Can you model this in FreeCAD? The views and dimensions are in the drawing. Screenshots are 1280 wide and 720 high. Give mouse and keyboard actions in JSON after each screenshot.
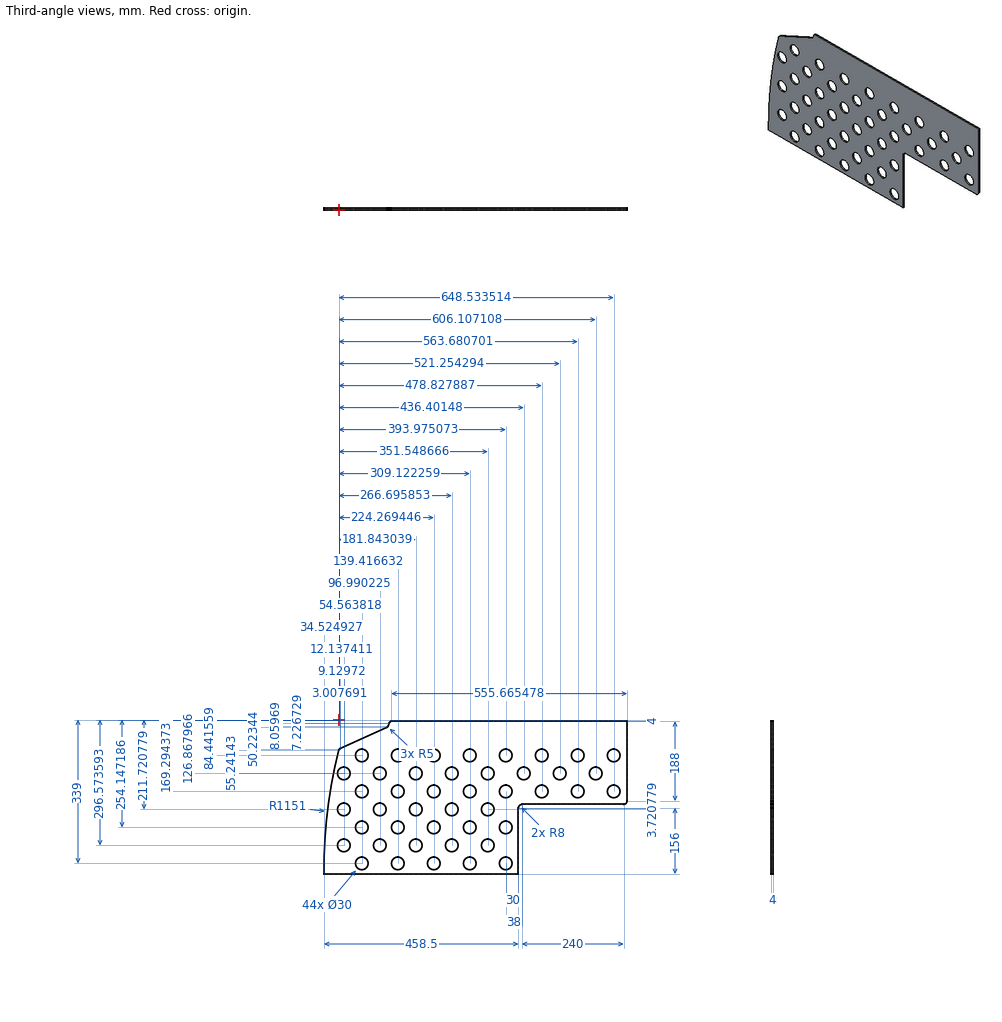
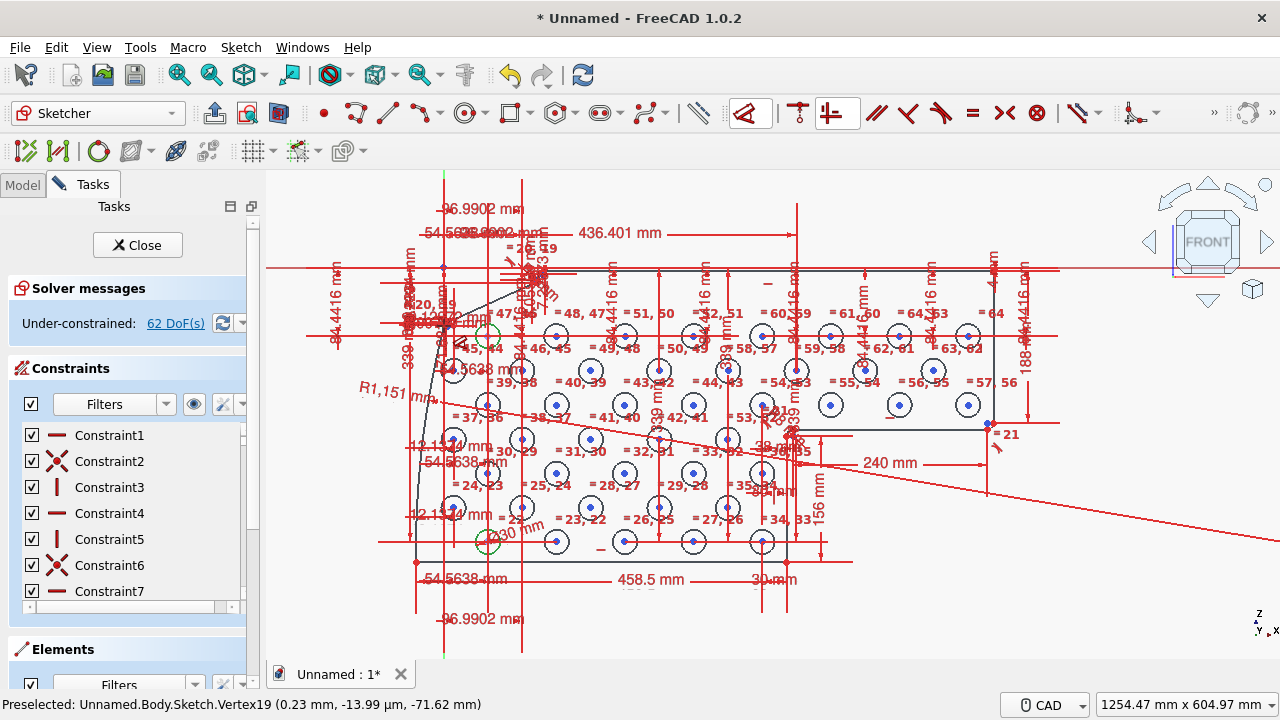
{"action": "left_click", "coordinate": [454, 371]}
{"action": "left_click", "coordinate": [410, 364]}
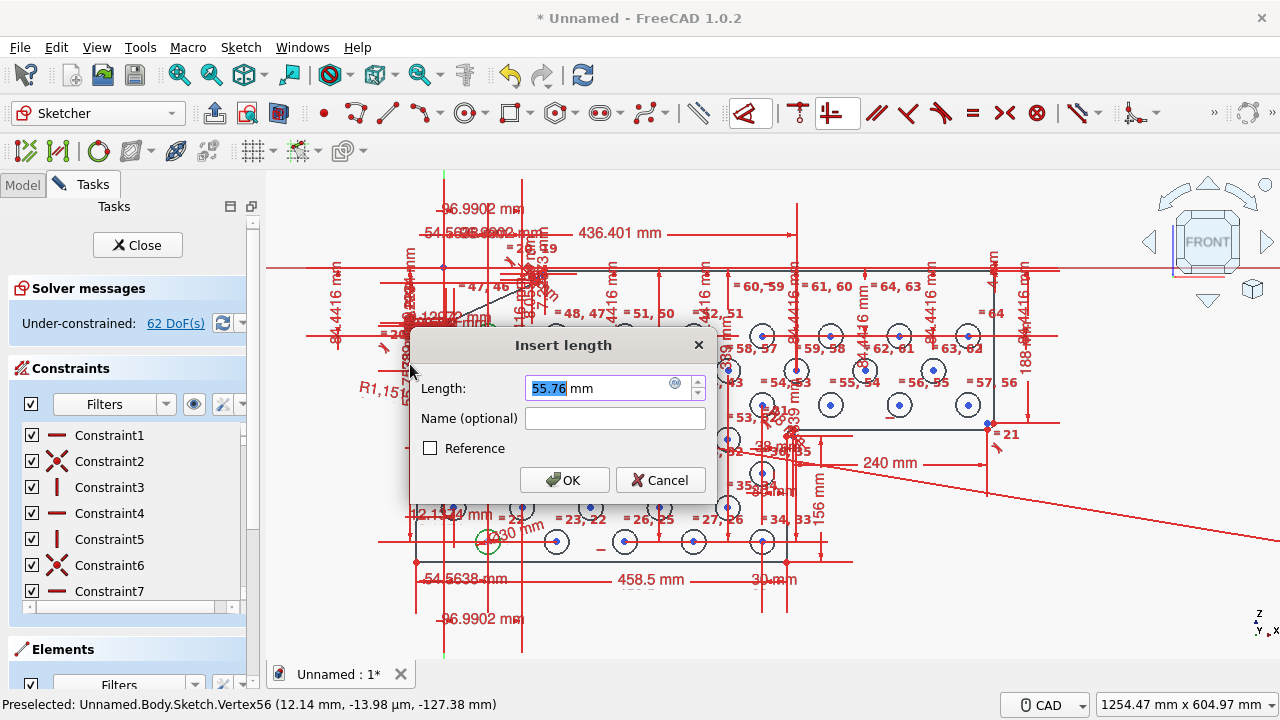
{"action": "type", "text": "55.24143"}
{"action": "key", "text": "Return"}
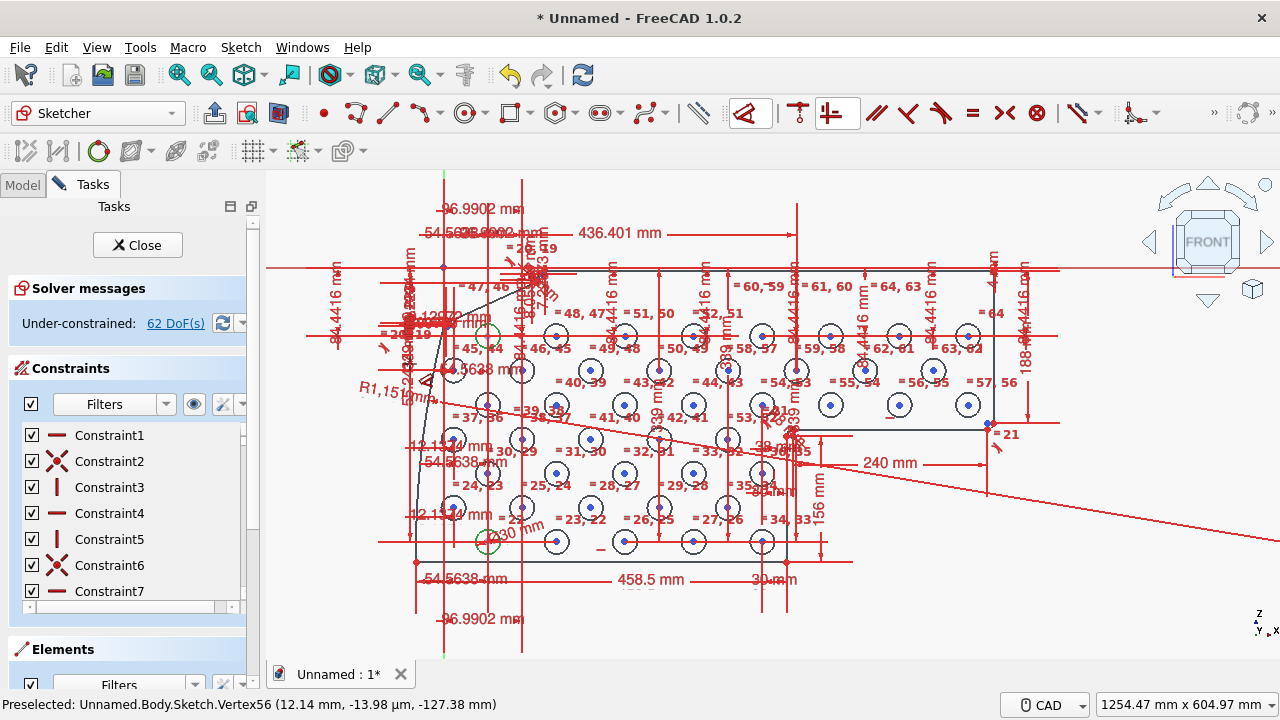
{"action": "scroll", "coordinate": [787, 436], "scroll_direction": "up", "scroll_amount": 13}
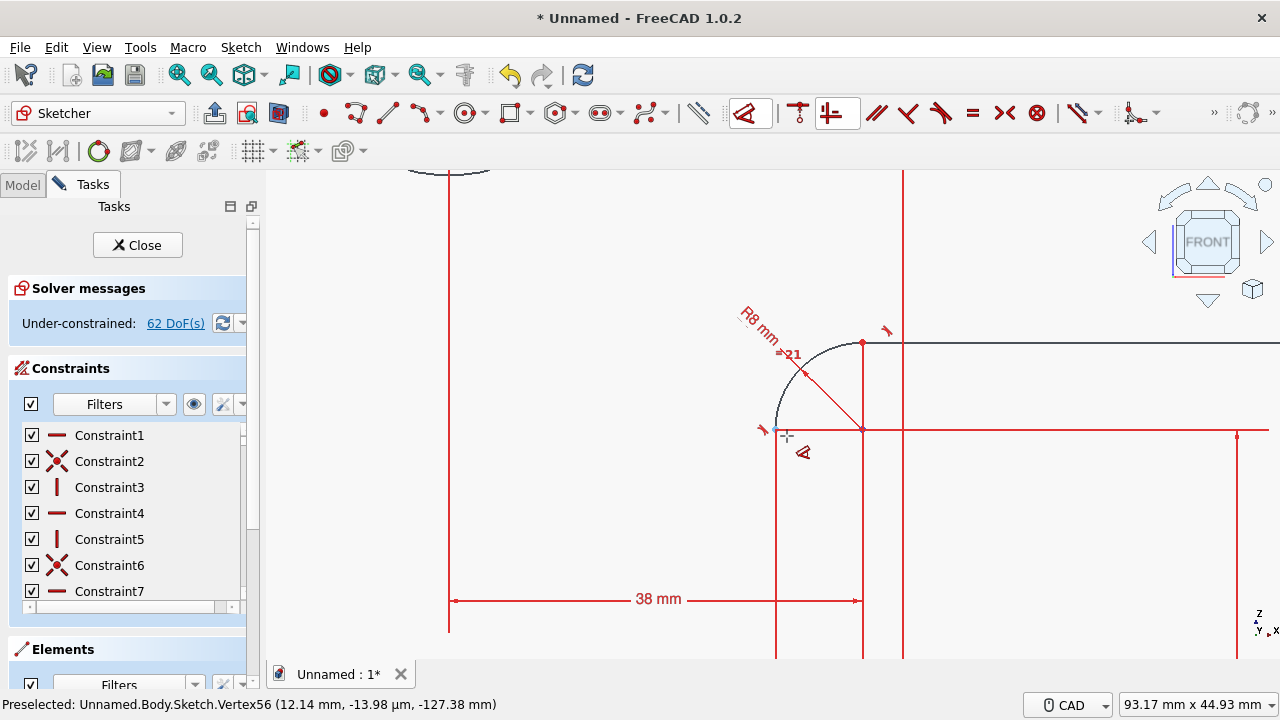
{"action": "left_click", "coordinate": [776, 430]}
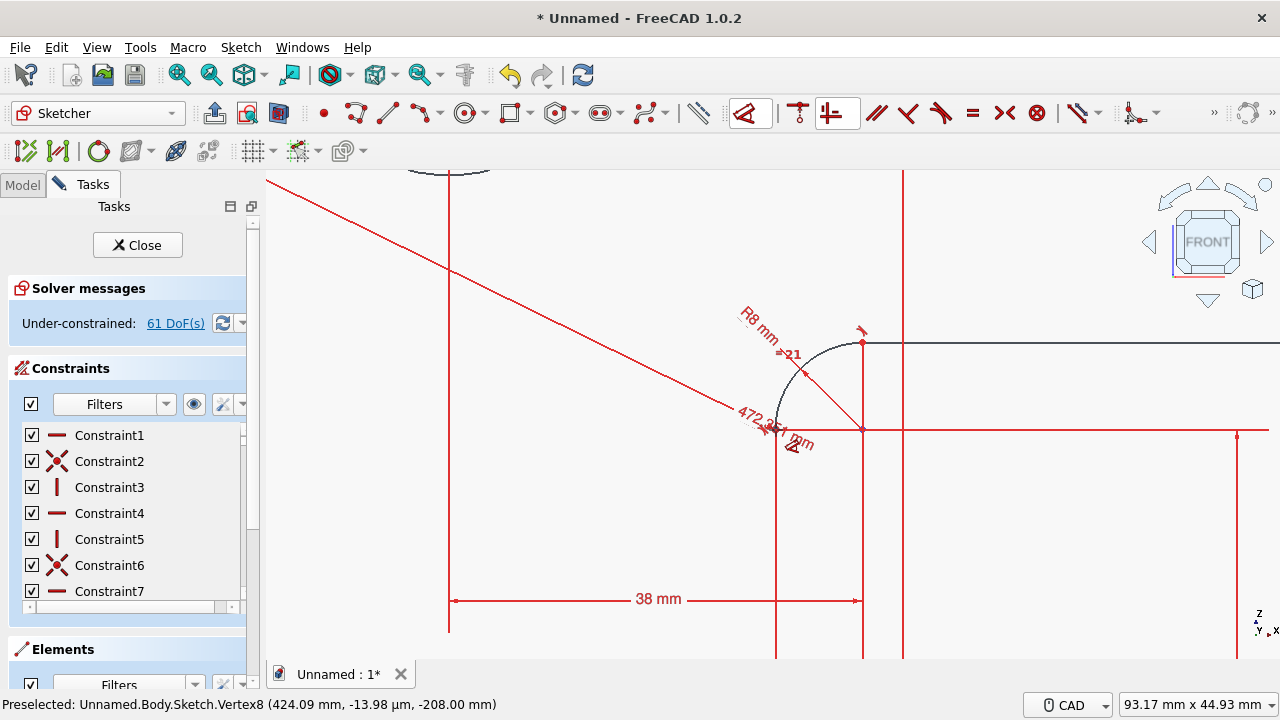
{"action": "scroll", "coordinate": [787, 436], "scroll_direction": "down", "scroll_amount": 13}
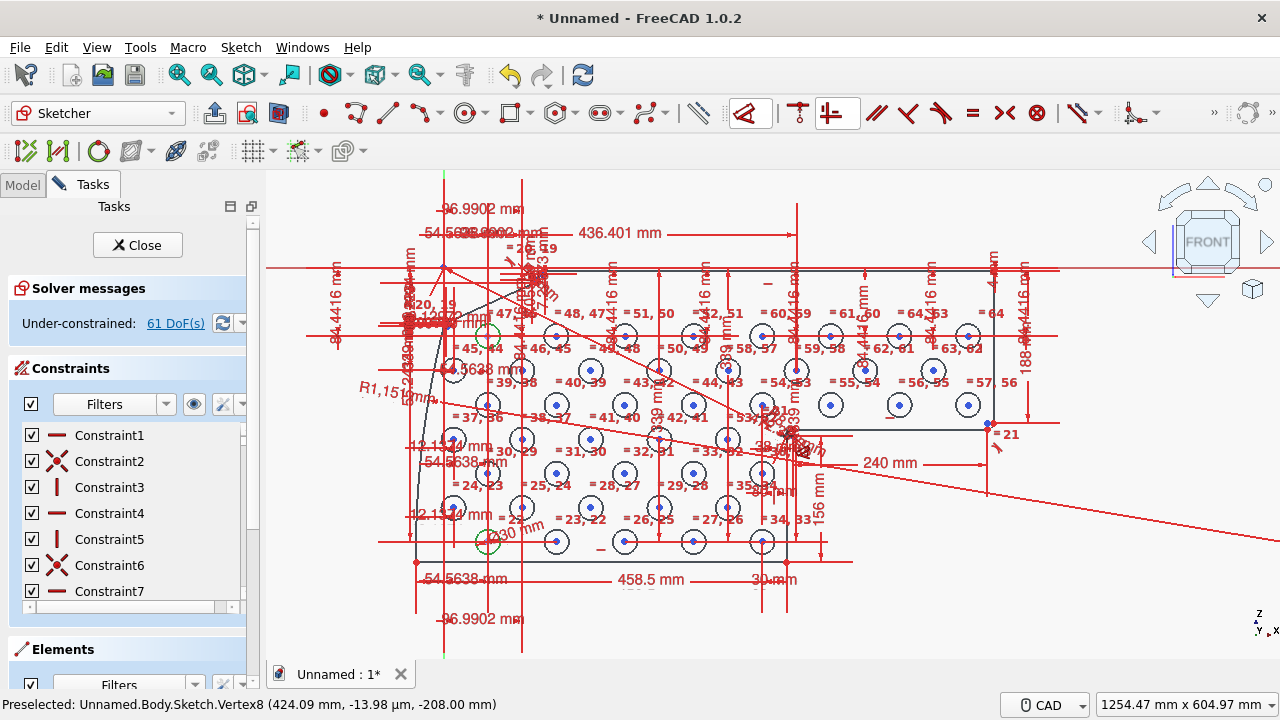
{"action": "scroll", "coordinate": [728, 440], "scroll_direction": "up", "scroll_amount": 13}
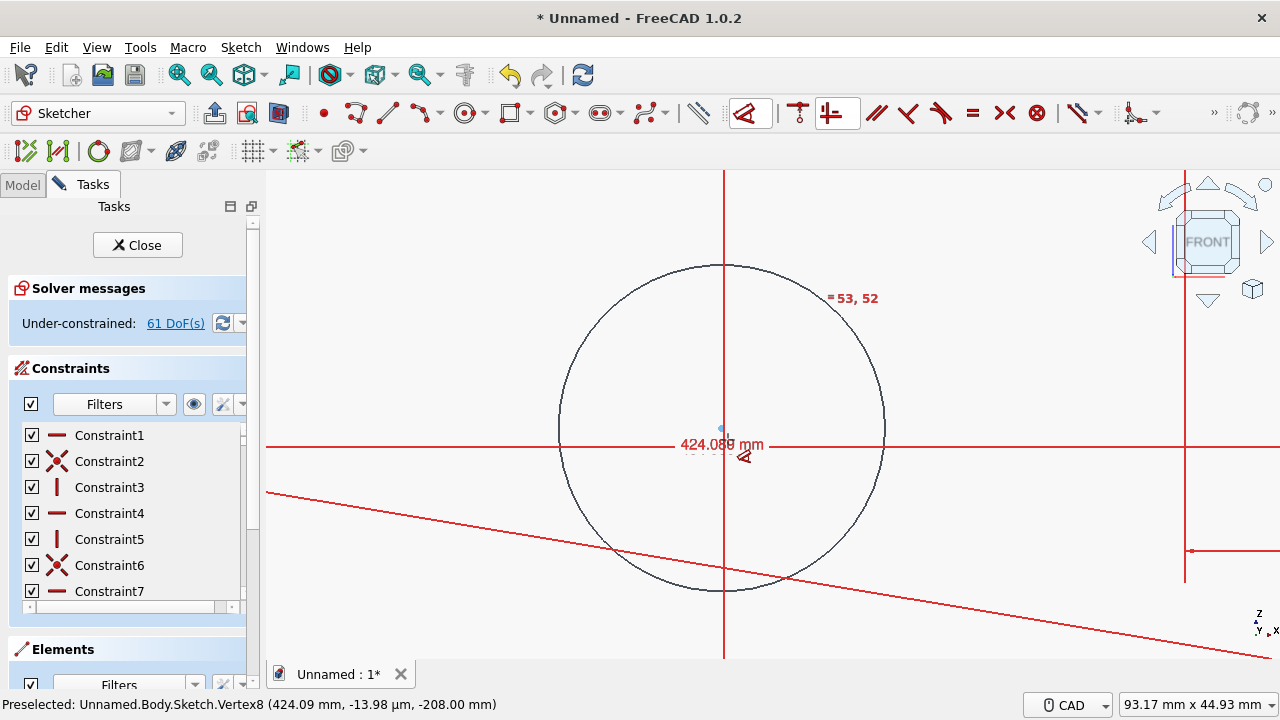
{"action": "left_click", "coordinate": [722, 428]}
{"action": "left_click", "coordinate": [688, 404]}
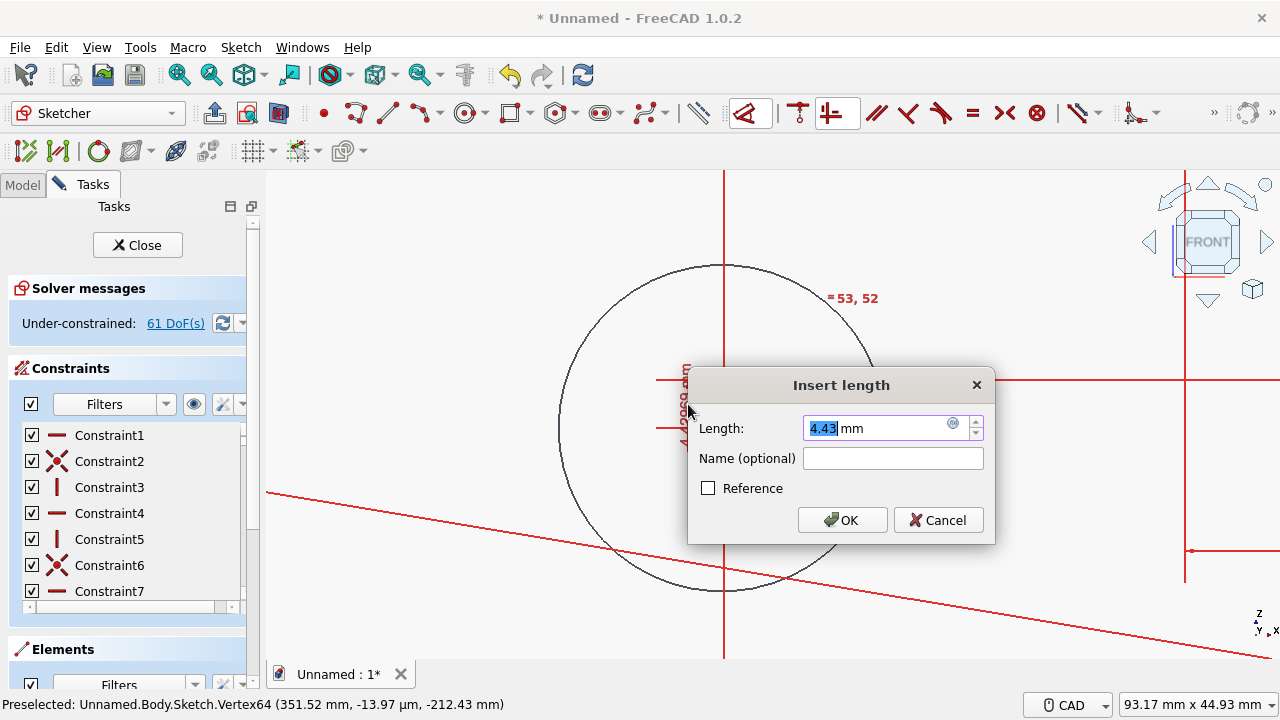
{"action": "type", "text": "3.720779"}
{"action": "key", "text": "Return"}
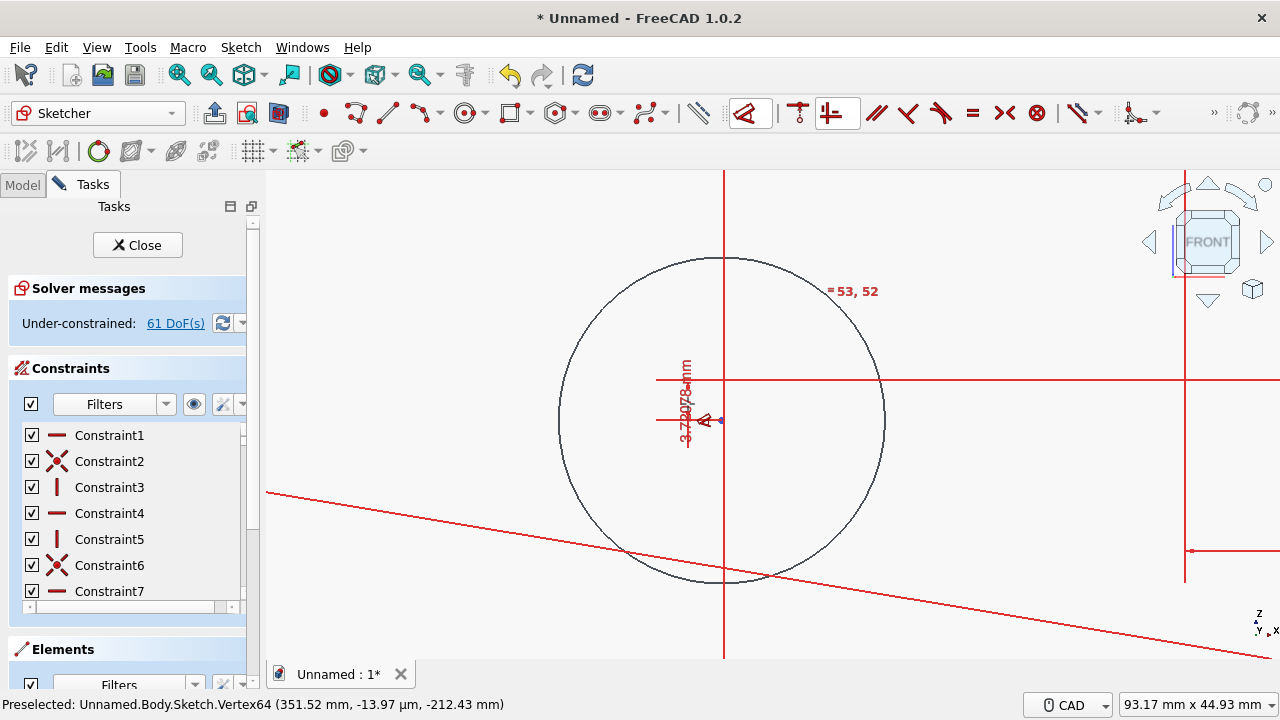
{"action": "scroll", "coordinate": [728, 440], "scroll_direction": "down", "scroll_amount": 13}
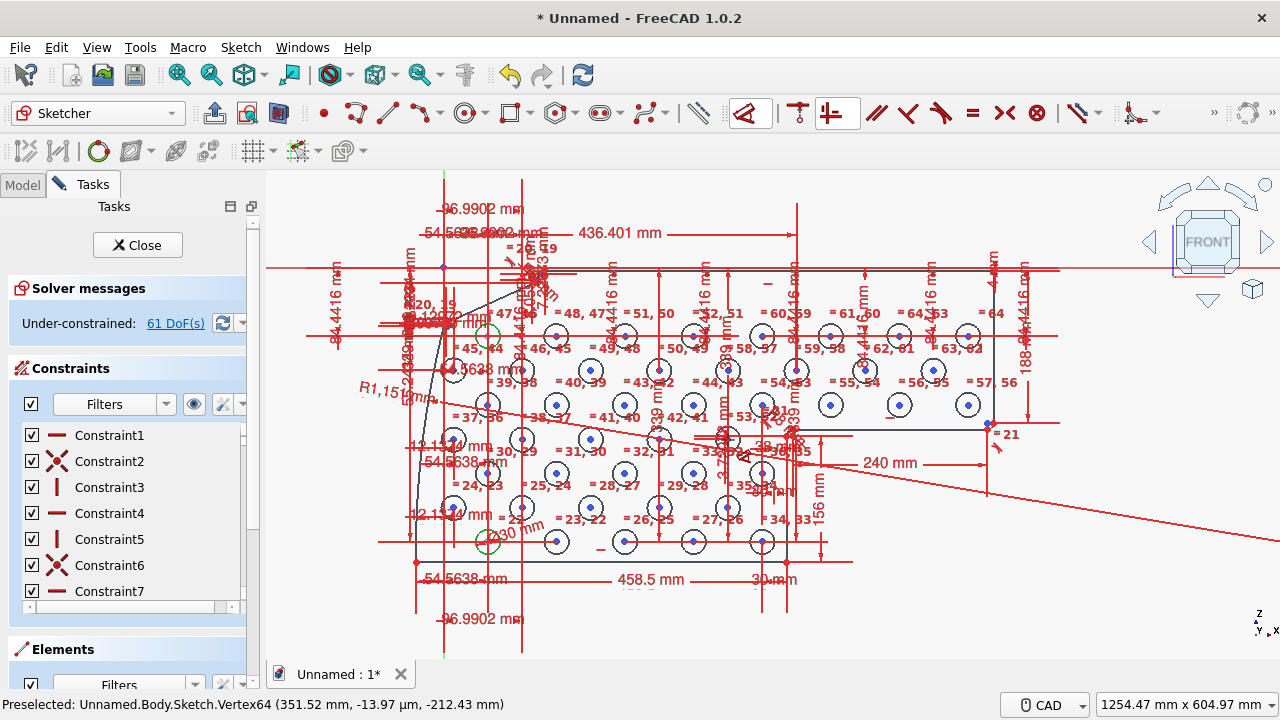
{"action": "scroll", "coordinate": [859, 271], "scroll_direction": "up", "scroll_amount": 8}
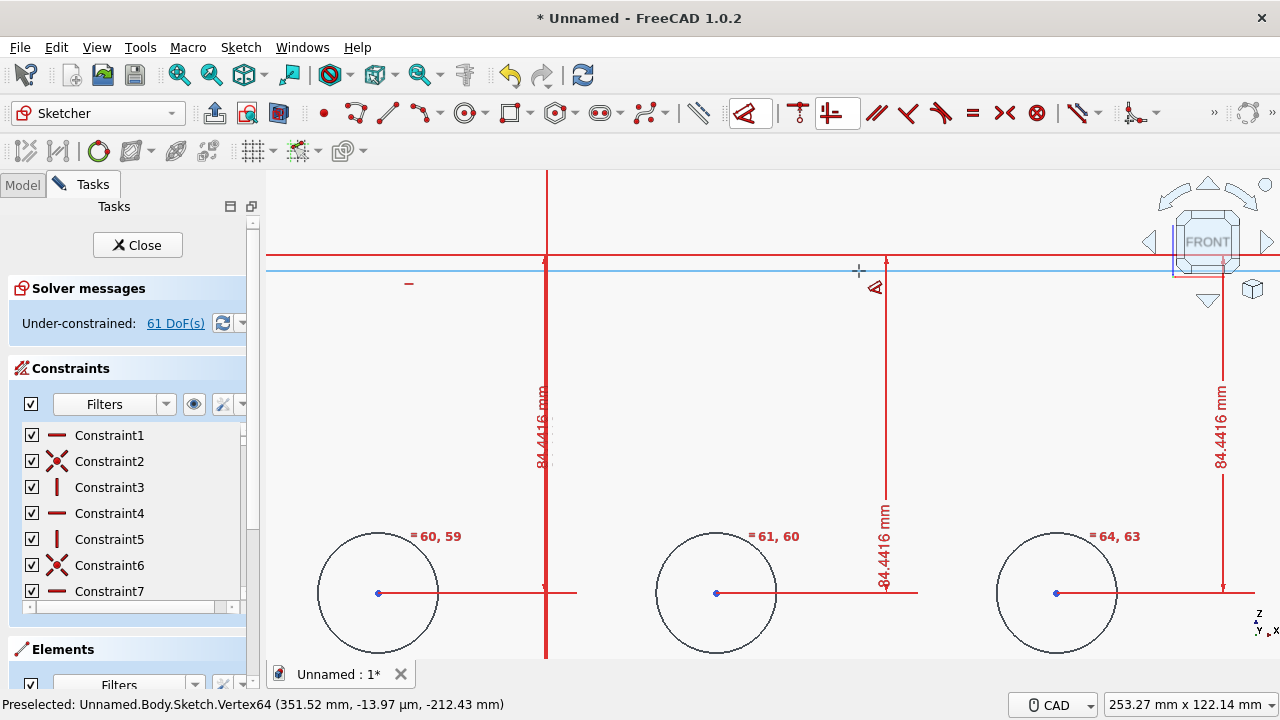
{"action": "left_click", "coordinate": [855, 271]}
{"action": "left_click", "coordinate": [704, 237]}